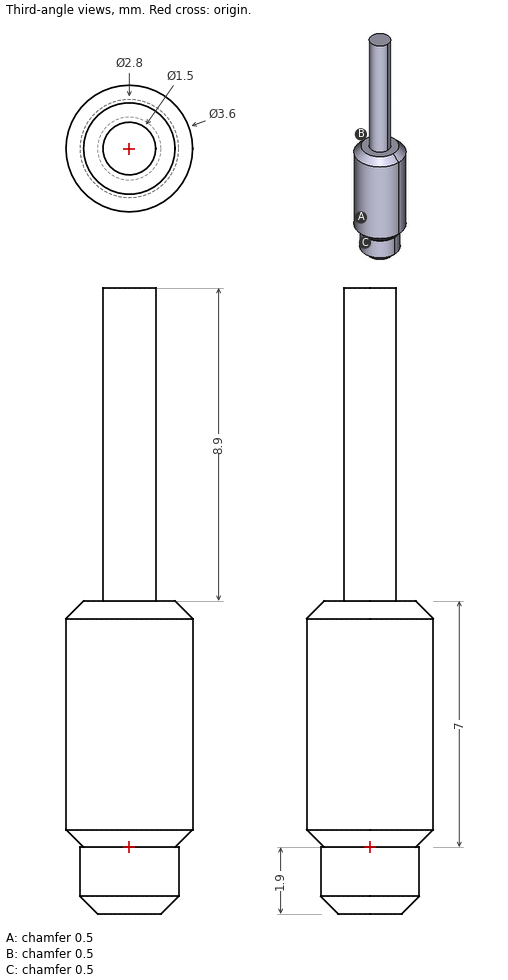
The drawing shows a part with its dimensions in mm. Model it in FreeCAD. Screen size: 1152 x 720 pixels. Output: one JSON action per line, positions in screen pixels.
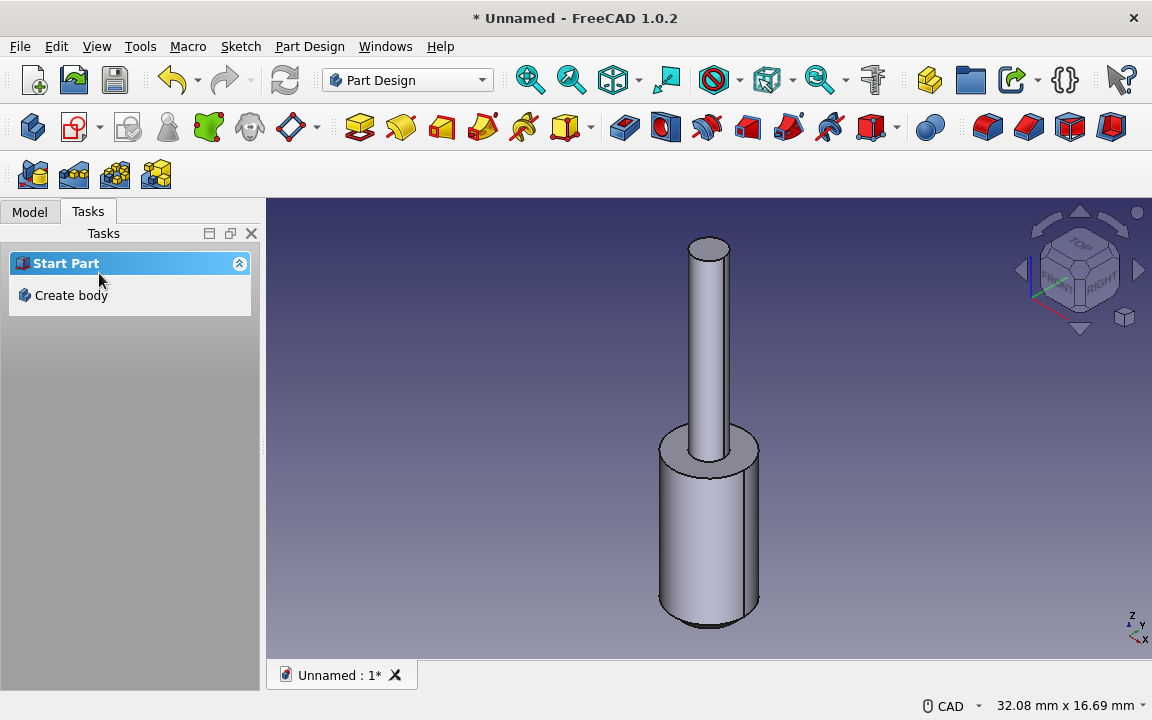
{"action": "left_click", "coordinate": [665, 462]}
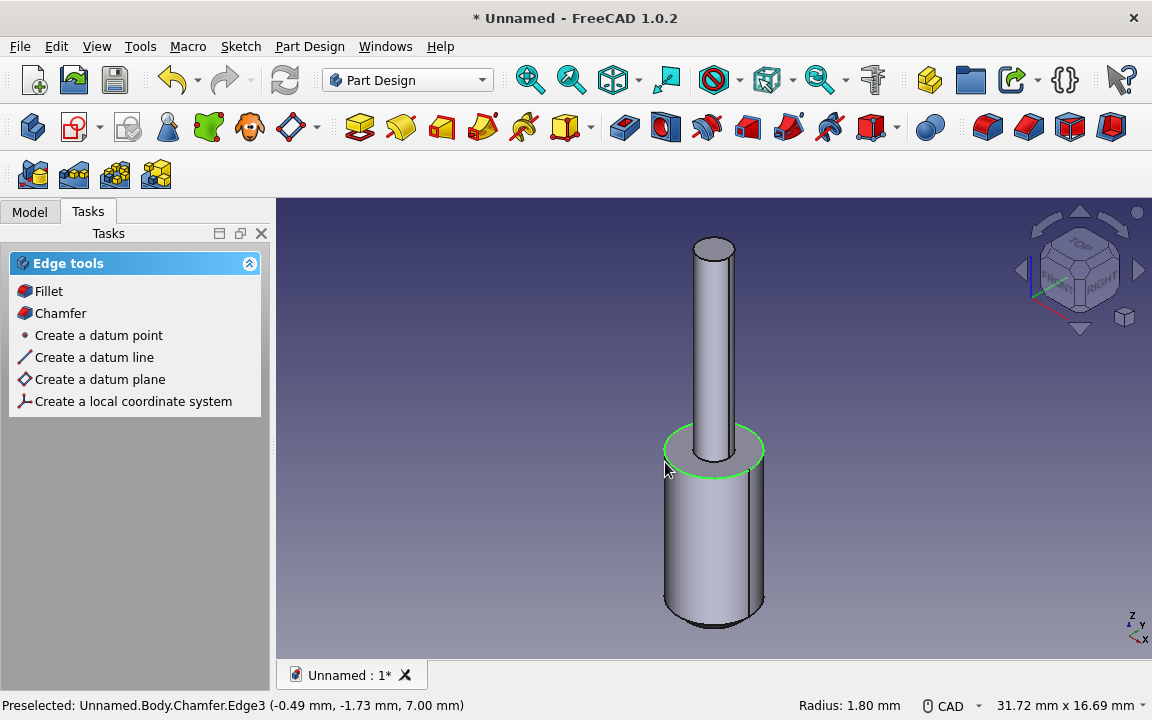
{"action": "left_click", "coordinate": [1029, 128]}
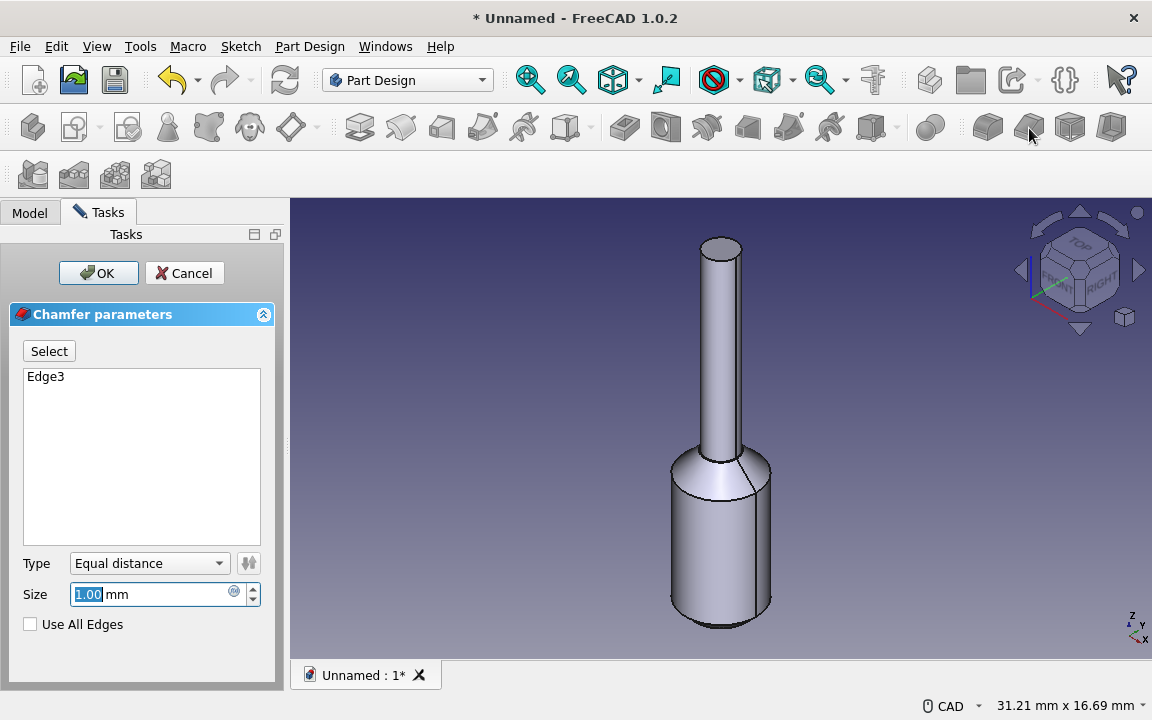
{"action": "type", "text": "0.5"}
{"action": "key", "text": "Tab"}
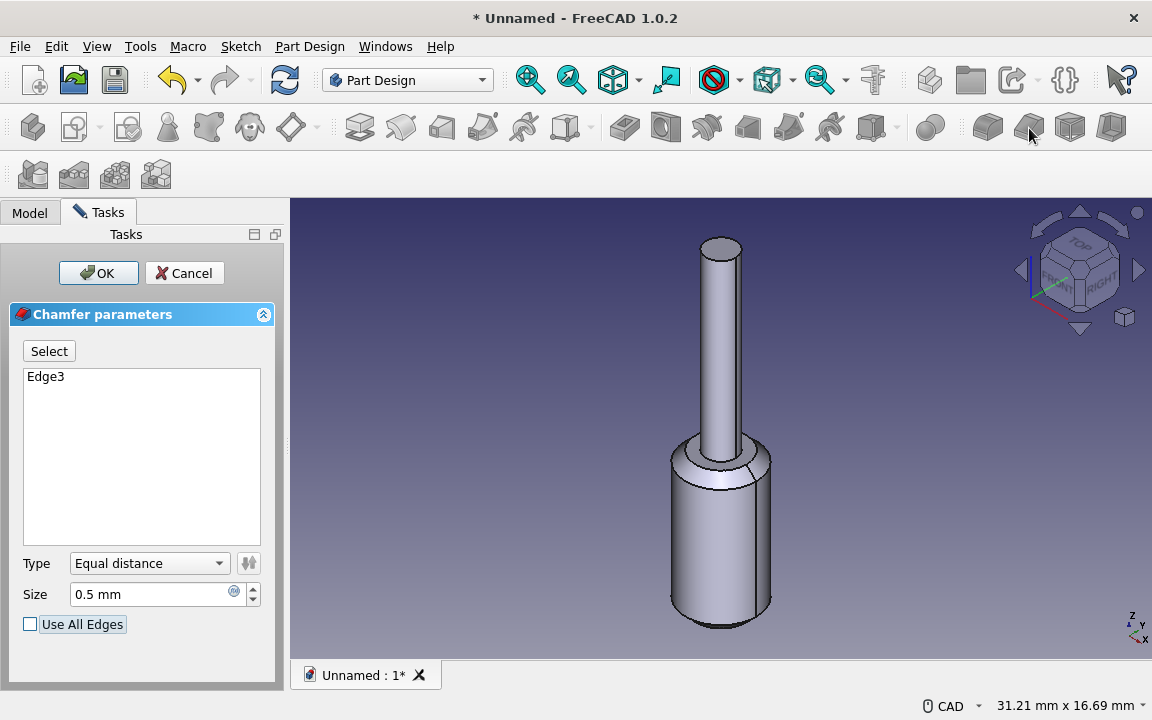
{"action": "left_click", "coordinate": [99, 273]}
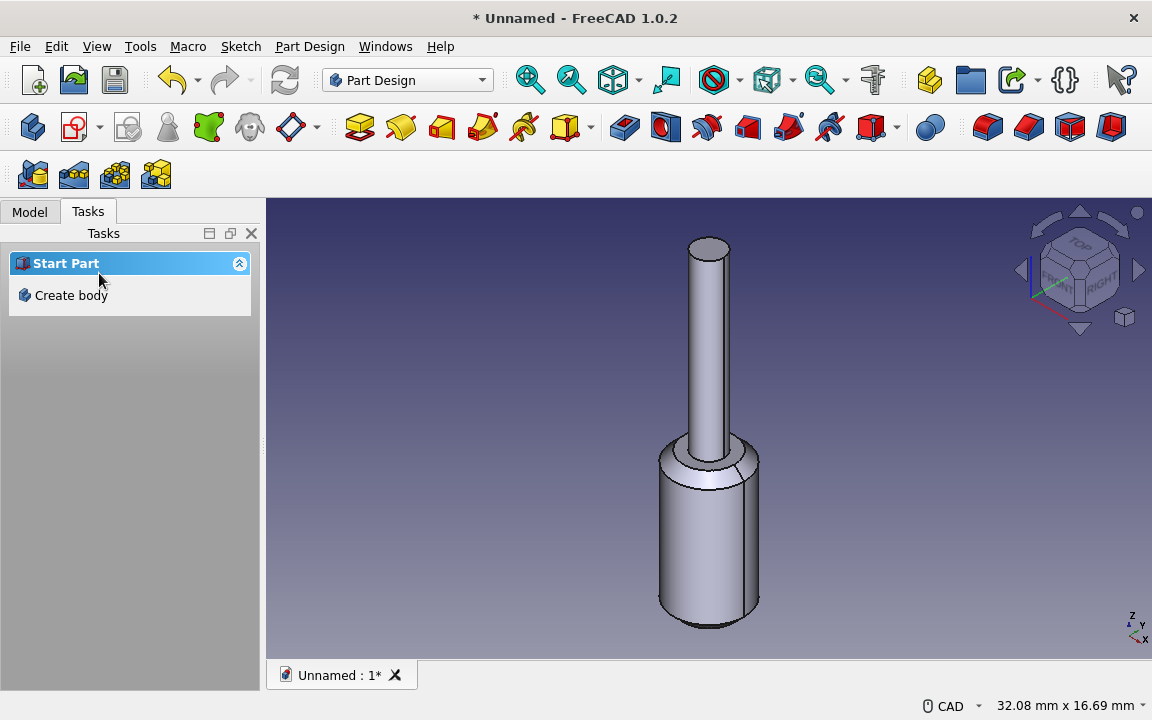
{"action": "key", "text": "5"}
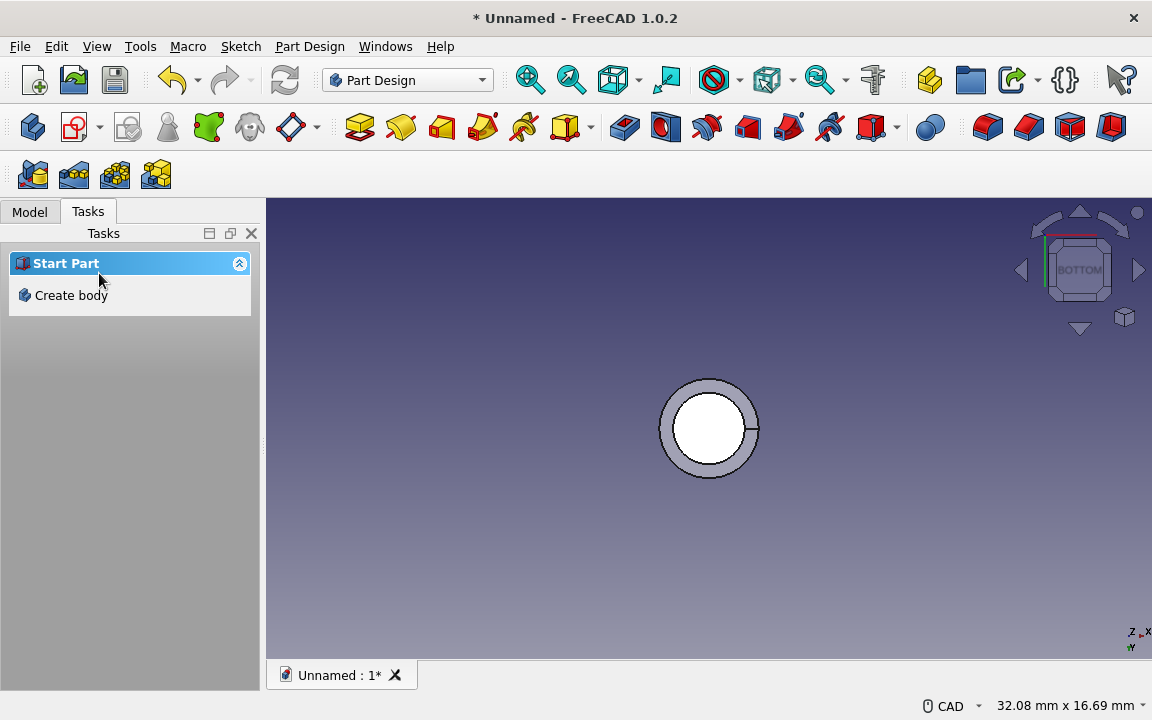
{"action": "key", "text": "v f"}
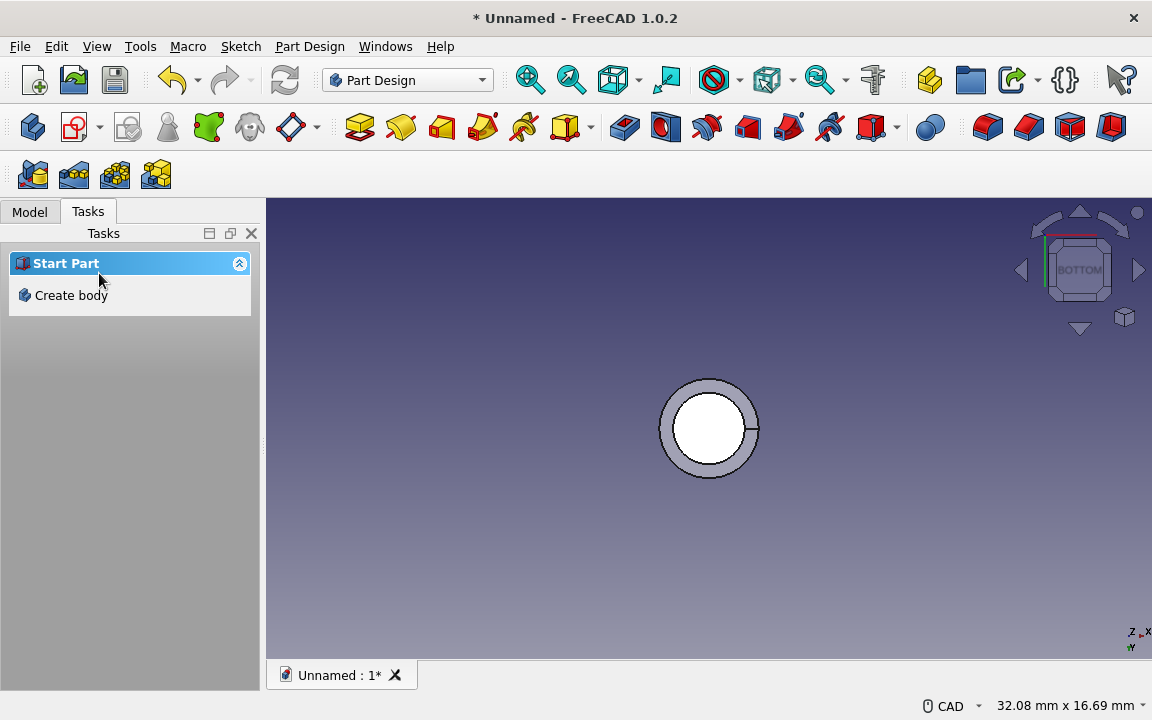
{"action": "left_click", "coordinate": [709, 427]}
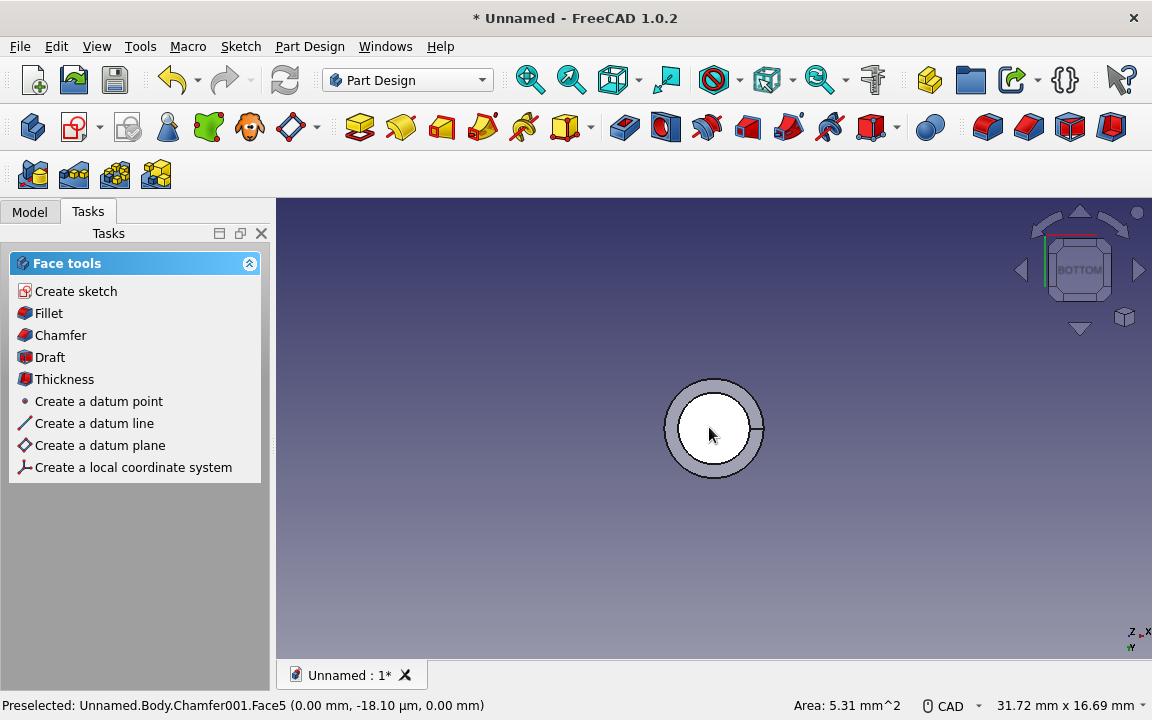
{"action": "left_click", "coordinate": [74, 128]}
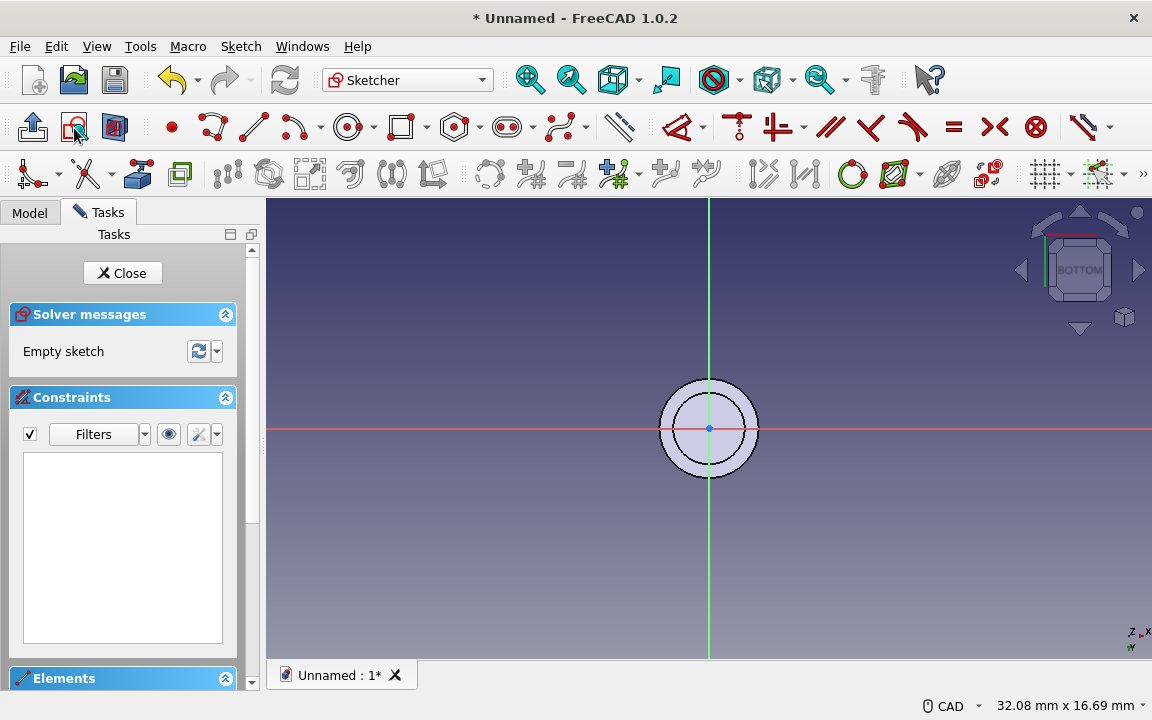
{"action": "scroll", "coordinate": [731, 429], "scroll_direction": "up", "scroll_amount": 7}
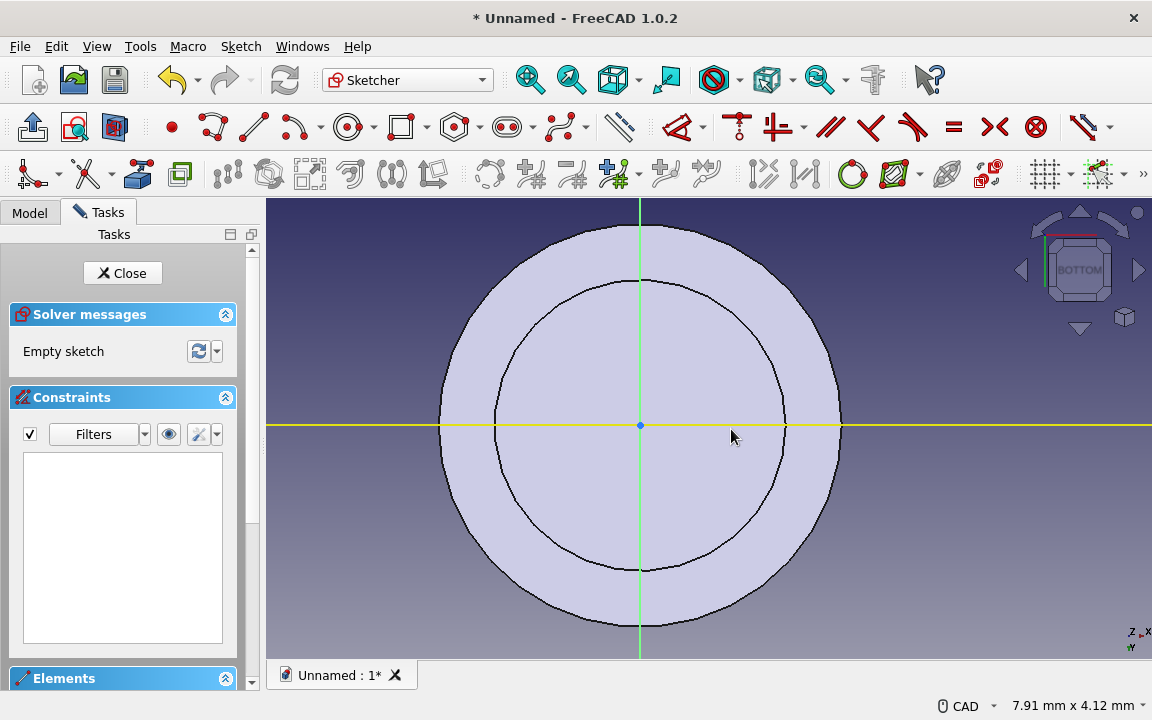
{"action": "key", "text": "g c"}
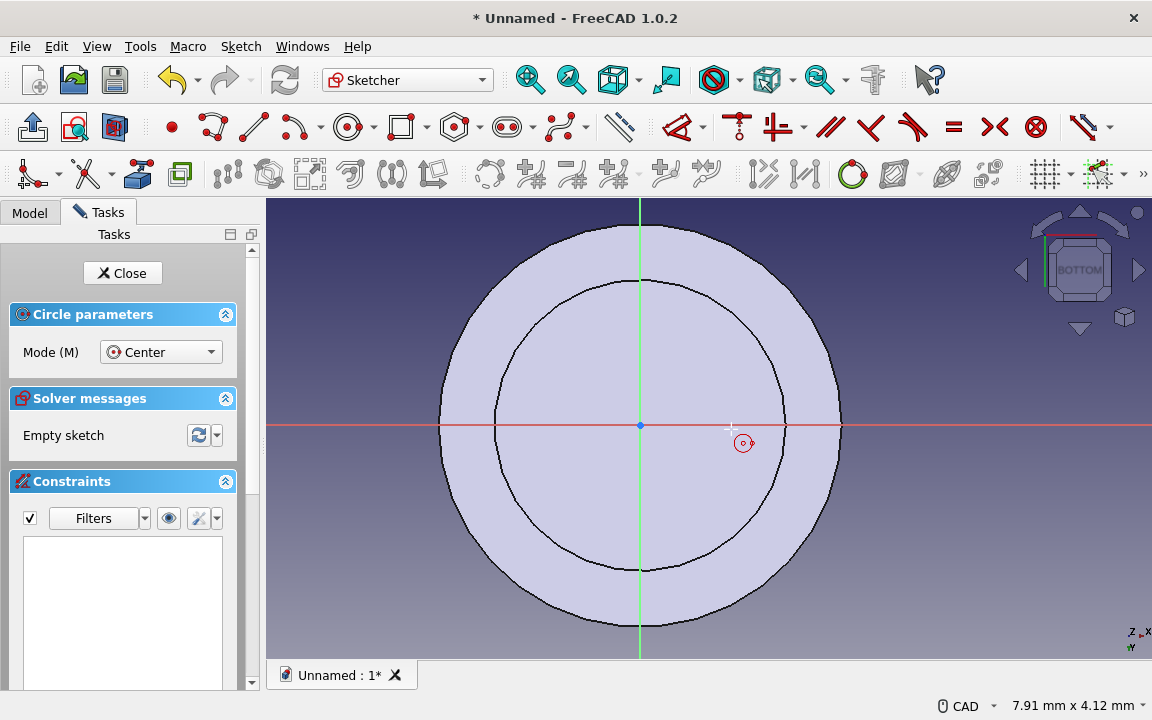
{"action": "left_click", "coordinate": [640, 425]}
{"action": "mouse_move", "coordinate": [751, 315]}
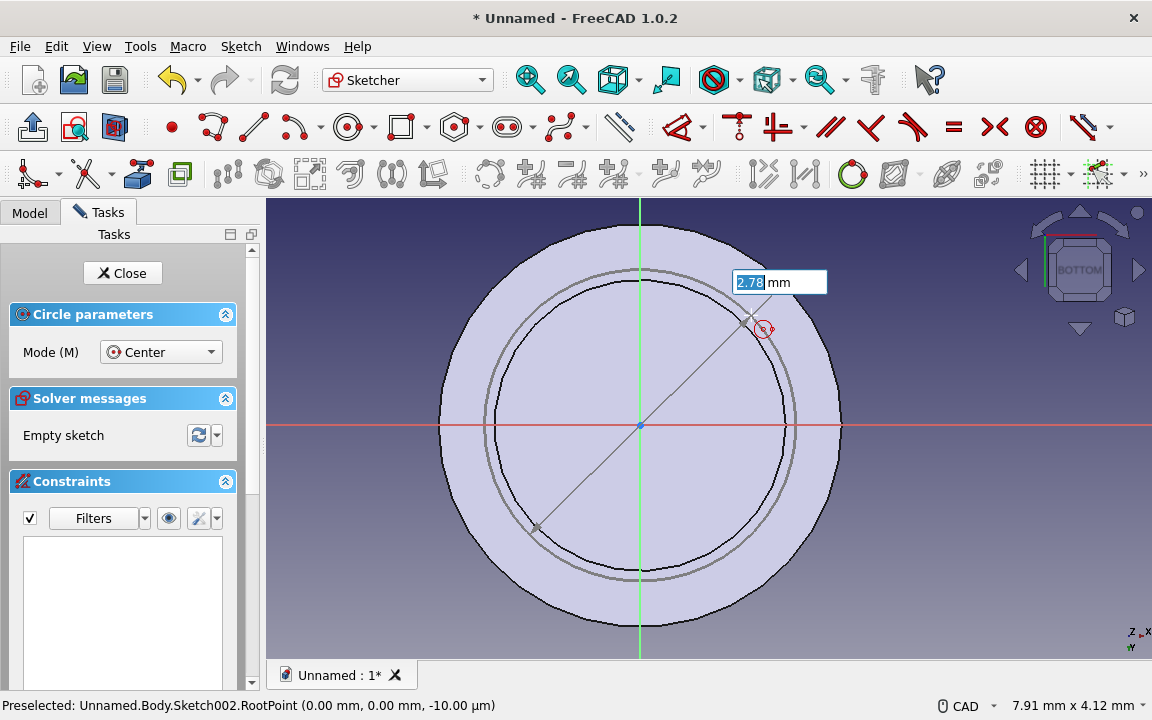
{"action": "type", "text": "2.8"}
{"action": "key", "text": "Return"}
{"action": "key", "text": "Escape"}